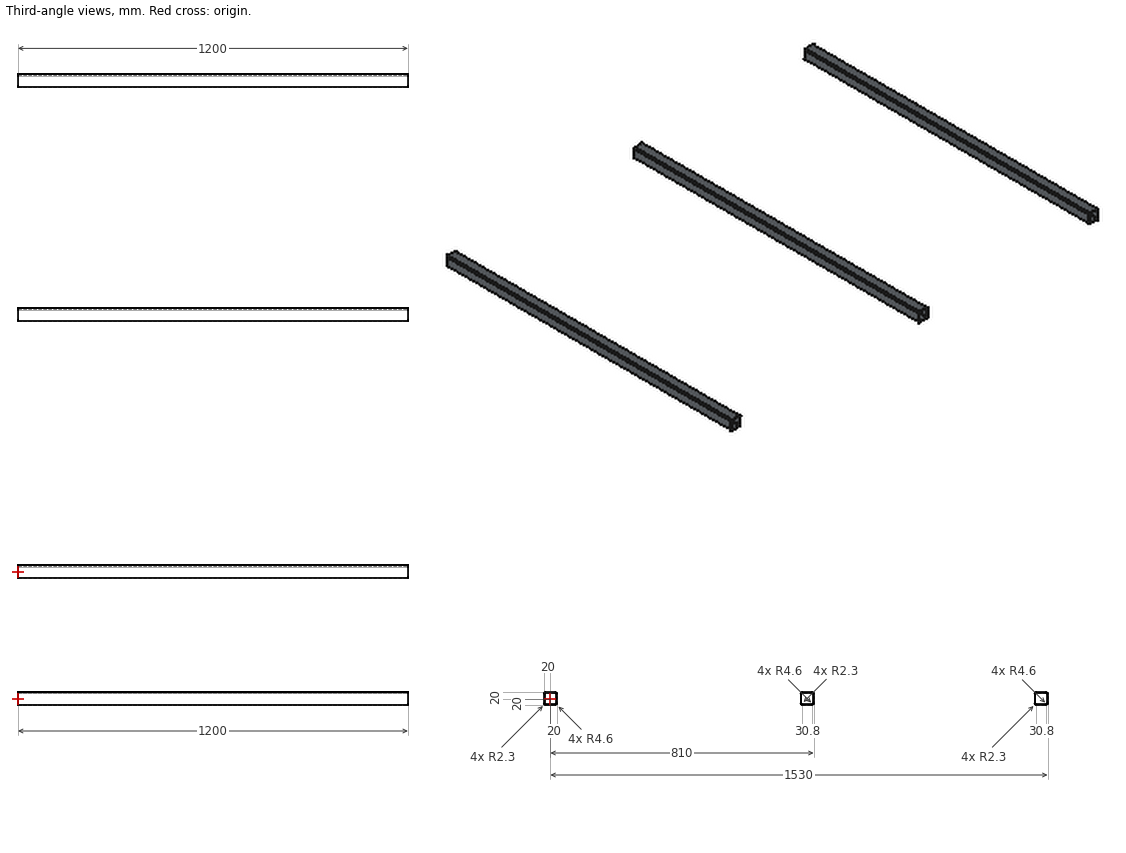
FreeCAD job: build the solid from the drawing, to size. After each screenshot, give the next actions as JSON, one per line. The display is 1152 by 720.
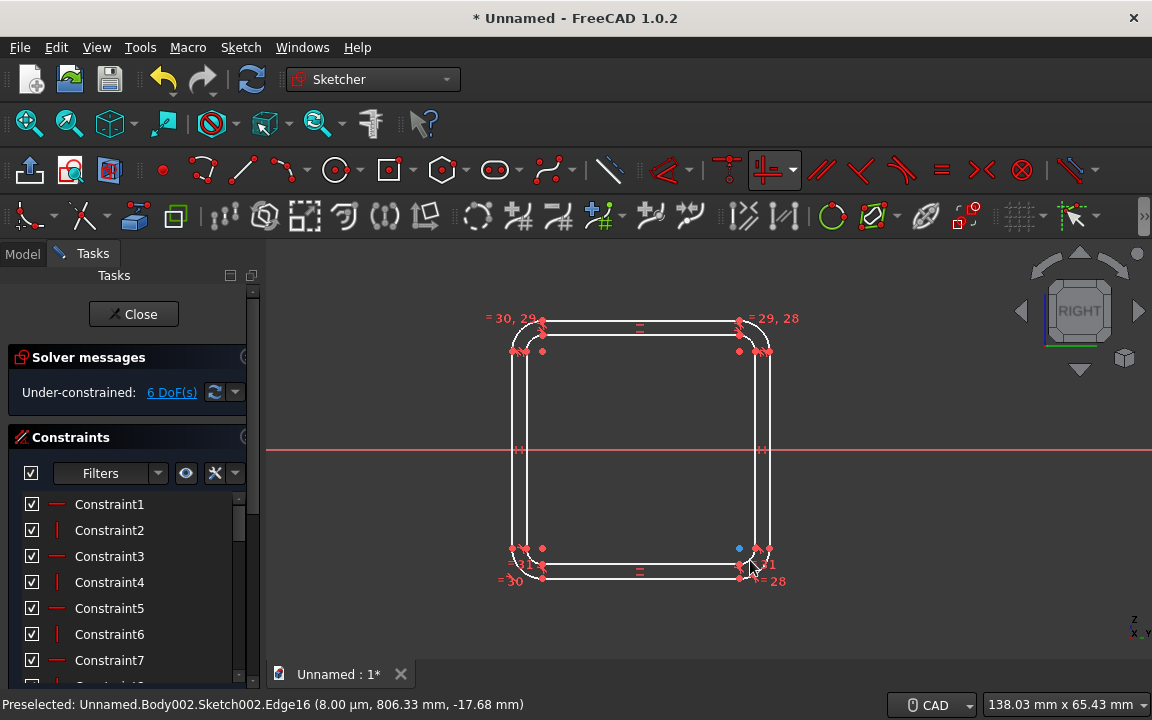
{"action": "key", "text": "d"}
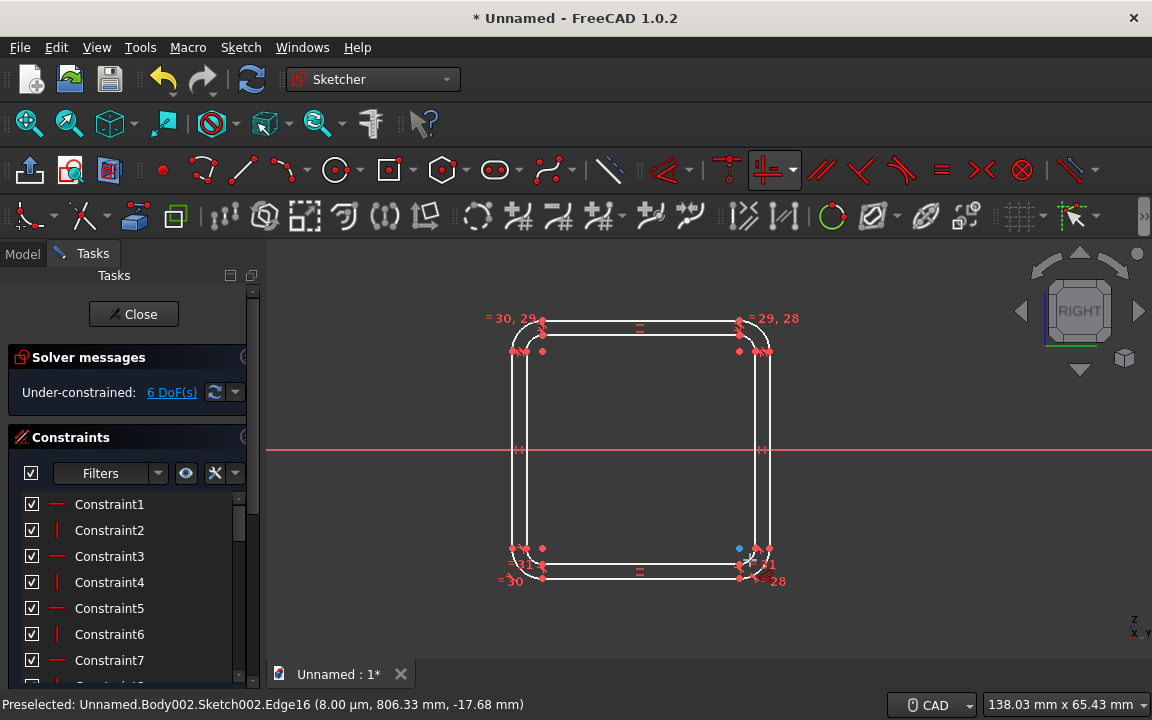
{"action": "scroll", "coordinate": [753, 575], "scroll_direction": "up", "scroll_amount": 2}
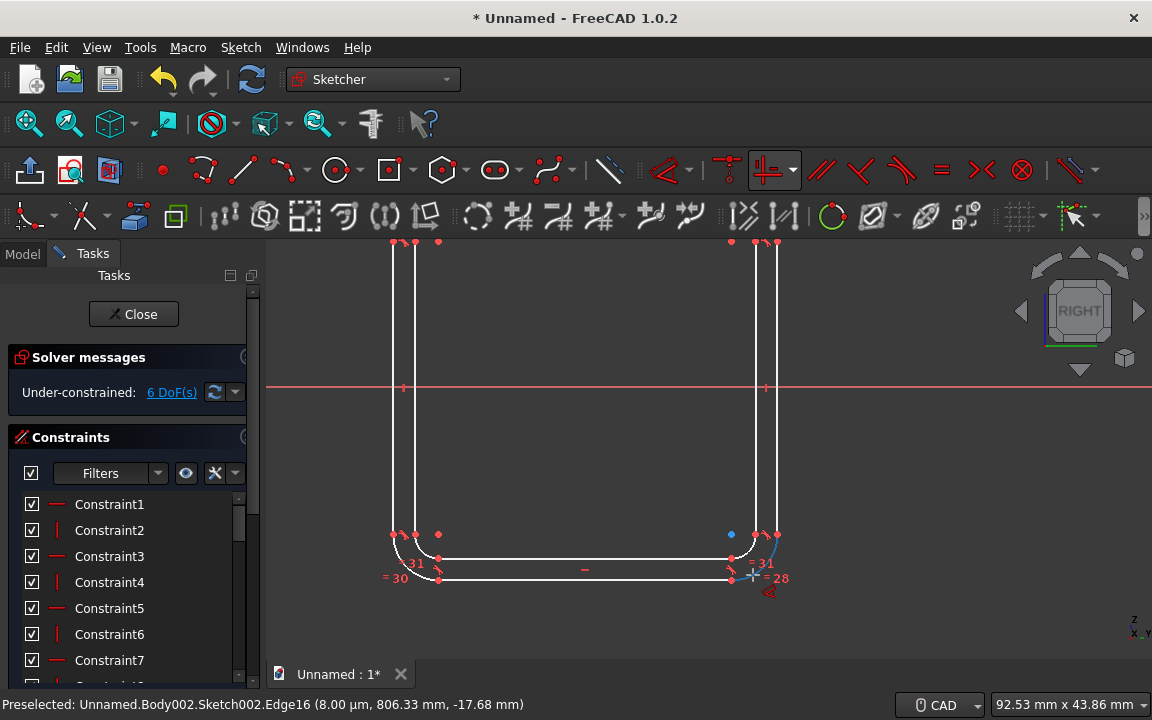
{"action": "left_click", "coordinate": [753, 575]}
{"action": "left_click", "coordinate": [768, 603]}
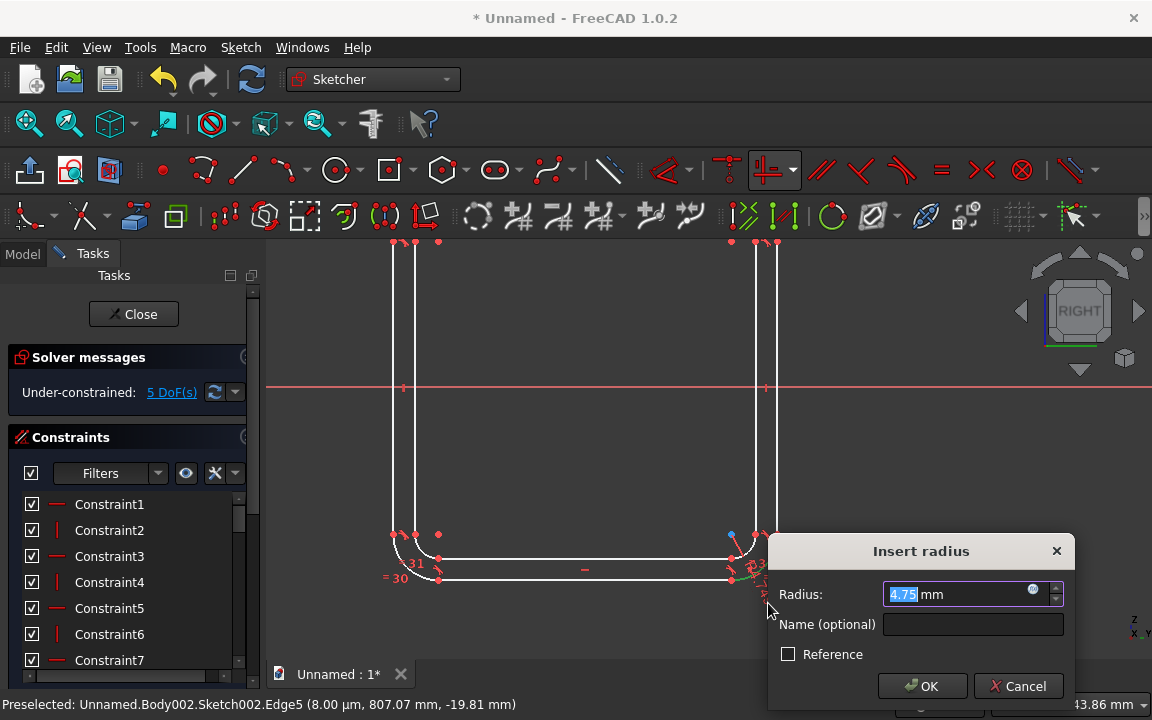
{"action": "type", "text": "4.6"}
{"action": "key", "text": "Return"}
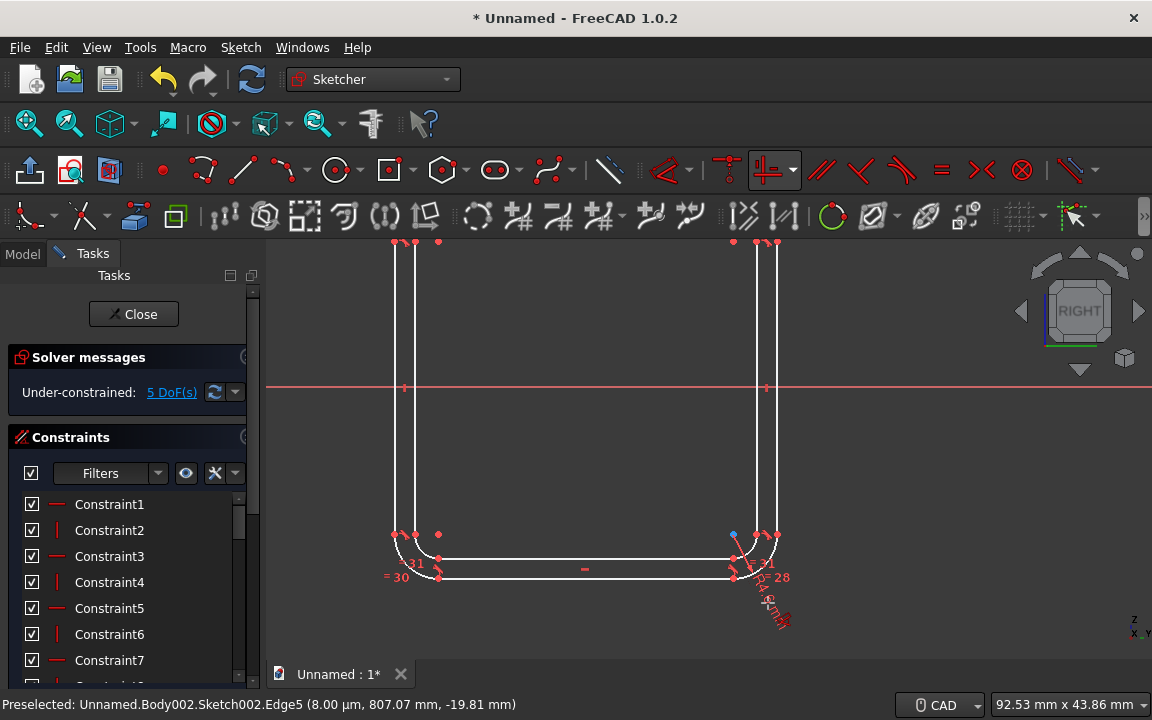
{"action": "scroll", "coordinate": [418, 546], "scroll_direction": "up", "scroll_amount": 3}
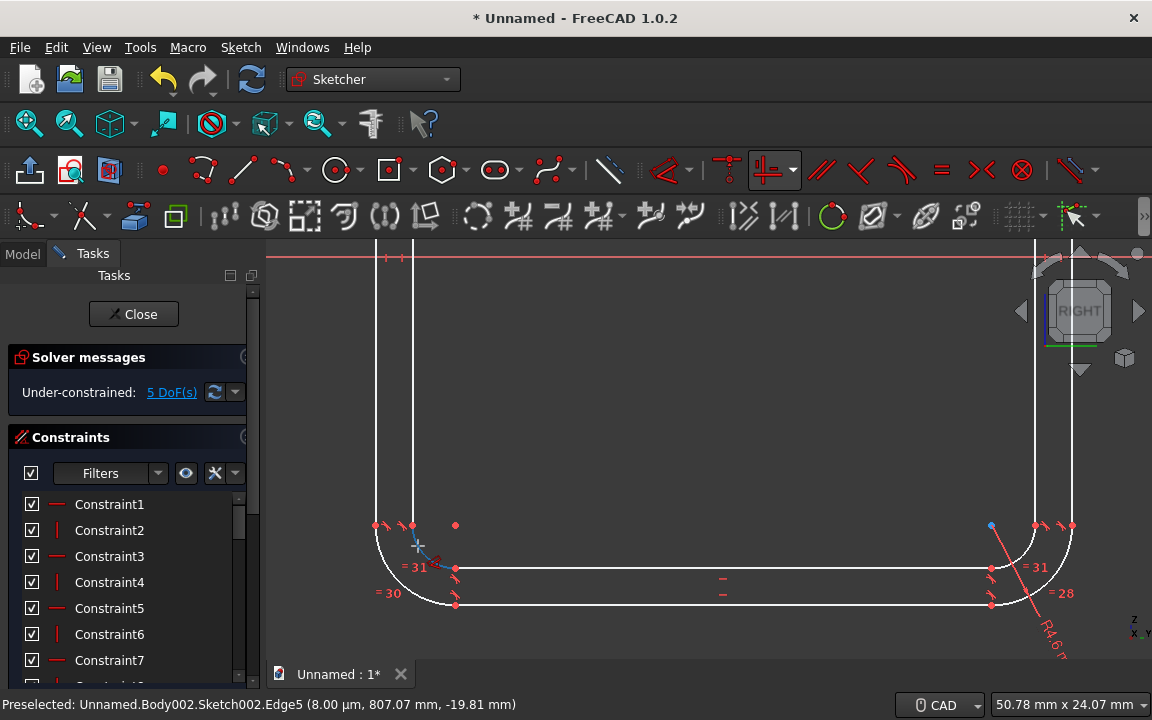
{"action": "left_click", "coordinate": [417, 545]}
{"action": "left_click", "coordinate": [390, 487]}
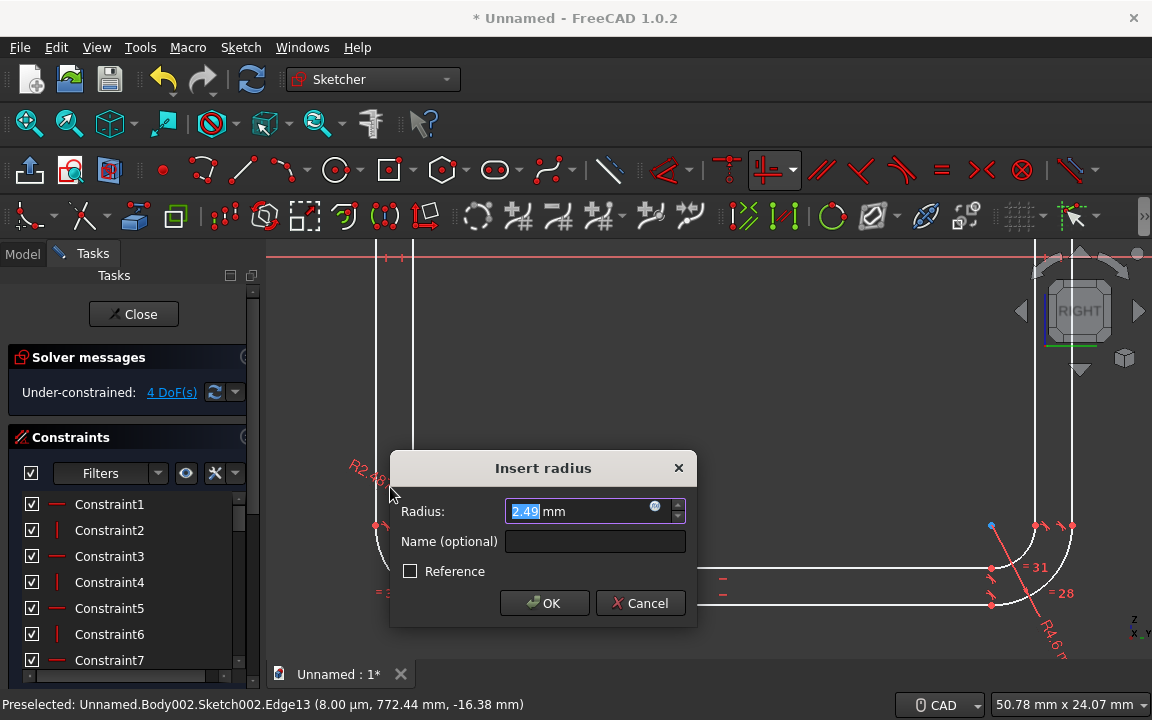
{"action": "type", "text": "2.3"}
{"action": "key", "text": "Return"}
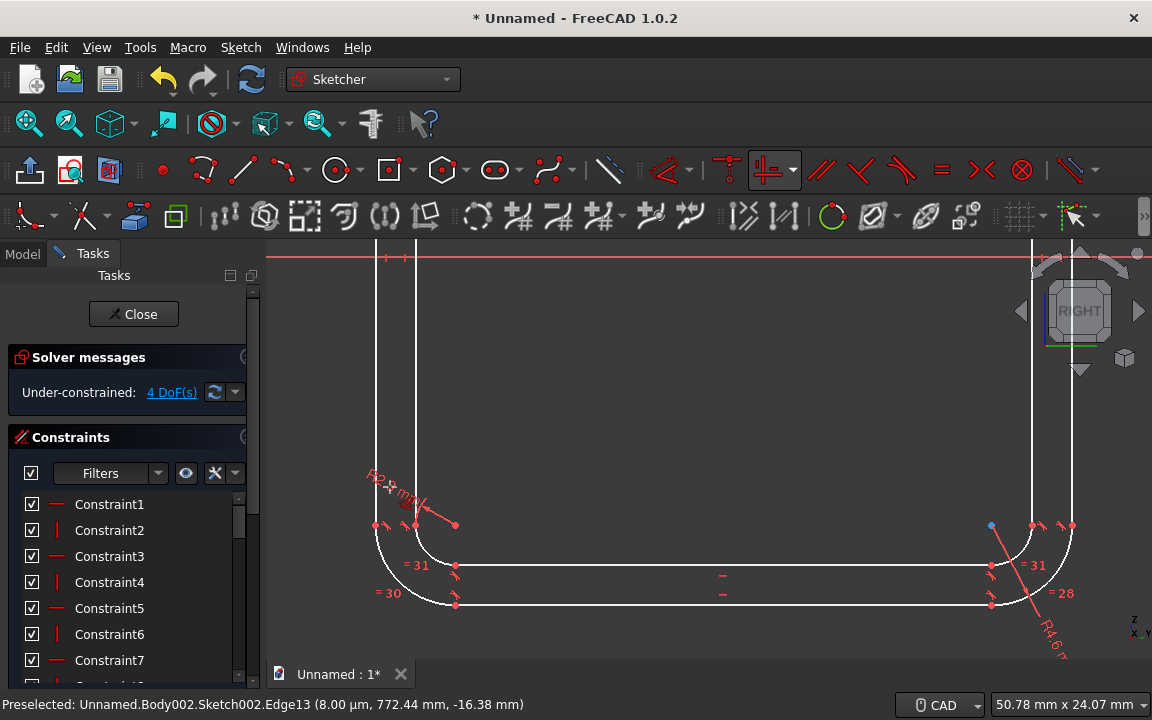
{"action": "left_click", "coordinate": [456, 605]}
{"action": "left_click", "coordinate": [490, 436]}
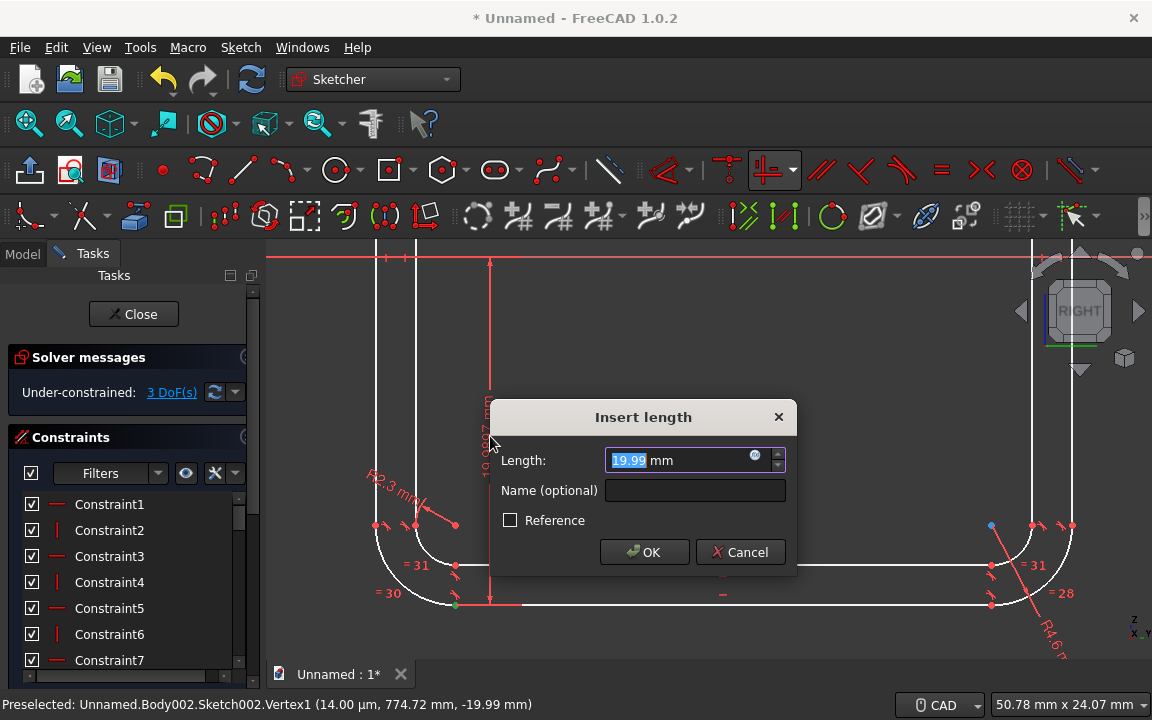
{"action": "type", "text": "20"}
{"action": "key", "text": "Return"}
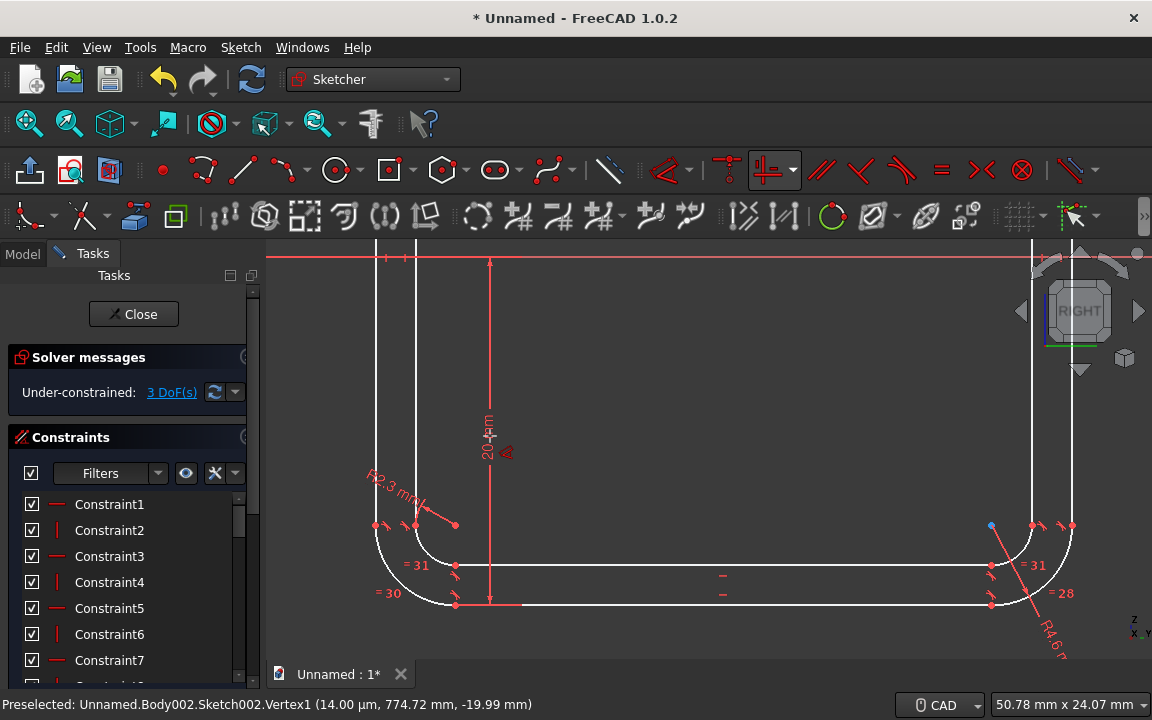
{"action": "scroll", "coordinate": [593, 561], "scroll_direction": "down", "scroll_amount": 5}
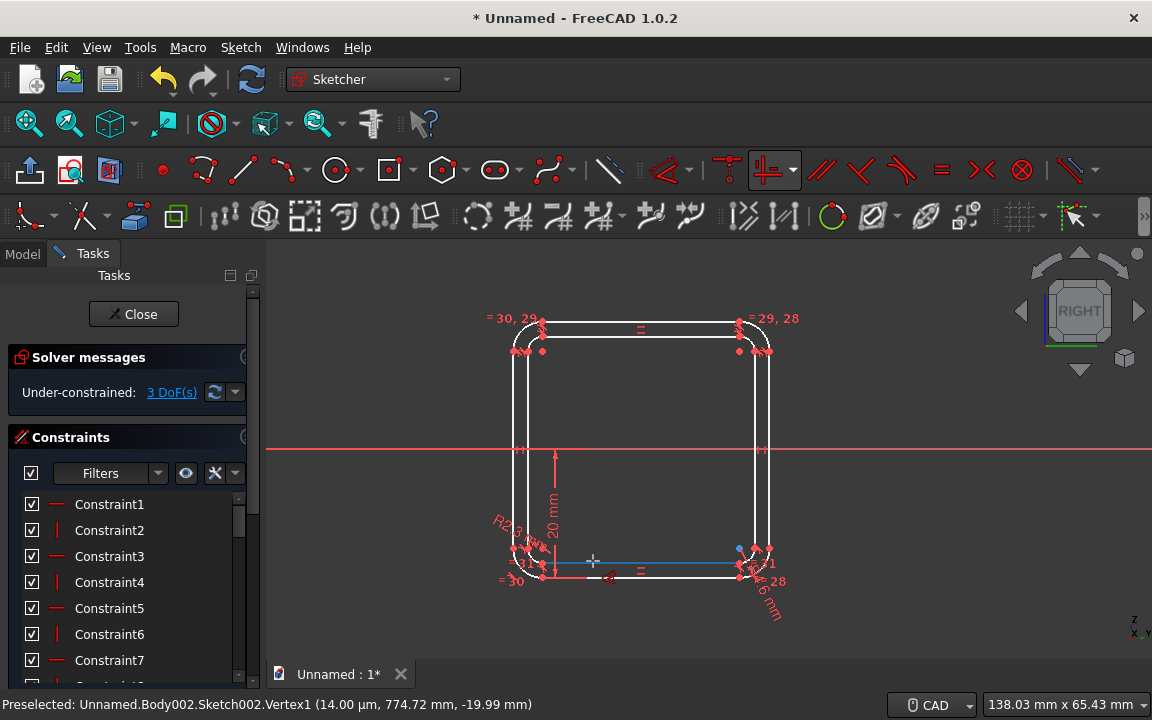
{"action": "left_click", "coordinate": [740, 322]}
{"action": "left_click", "coordinate": [798, 386]}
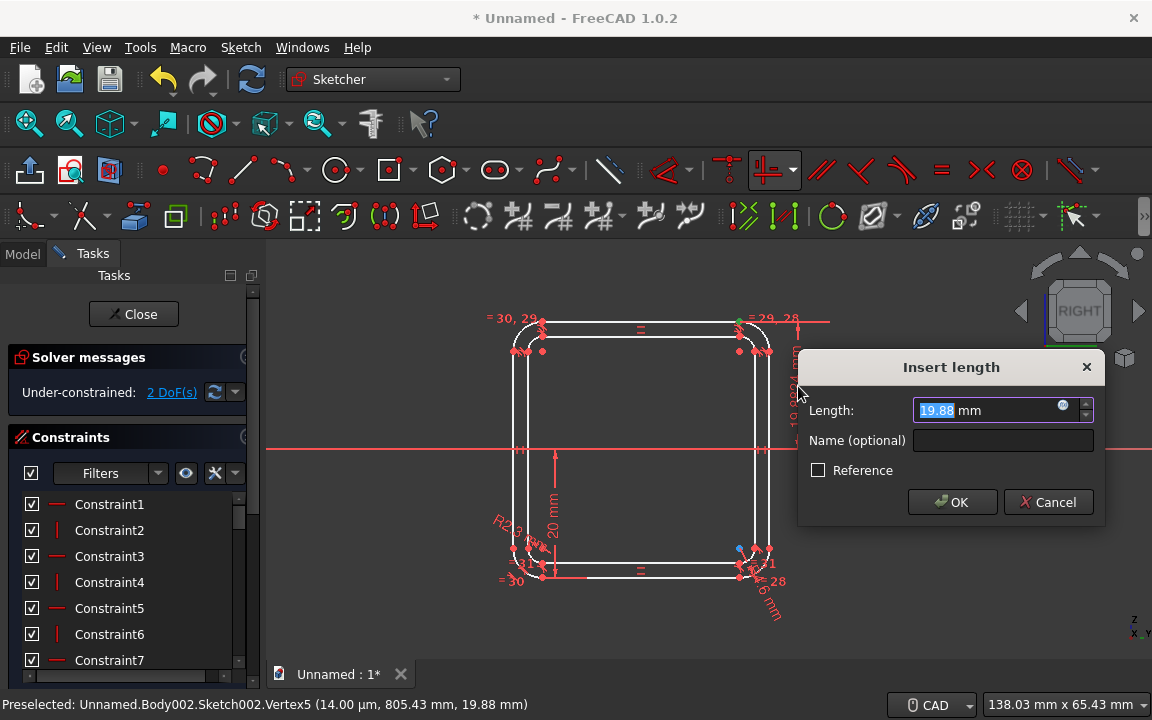
{"action": "type", "text": "20"}
{"action": "key", "text": "Return"}